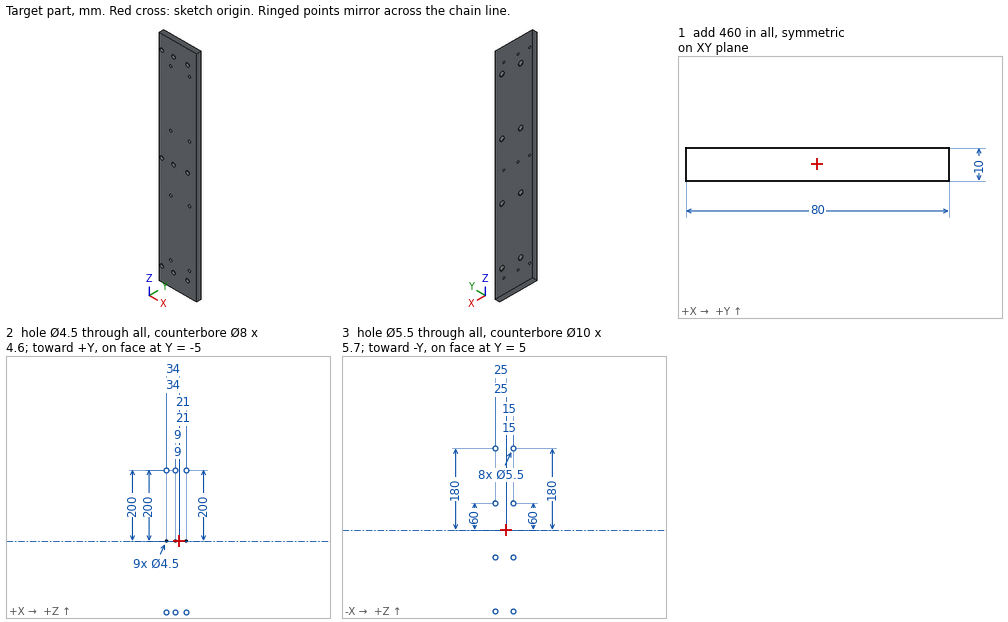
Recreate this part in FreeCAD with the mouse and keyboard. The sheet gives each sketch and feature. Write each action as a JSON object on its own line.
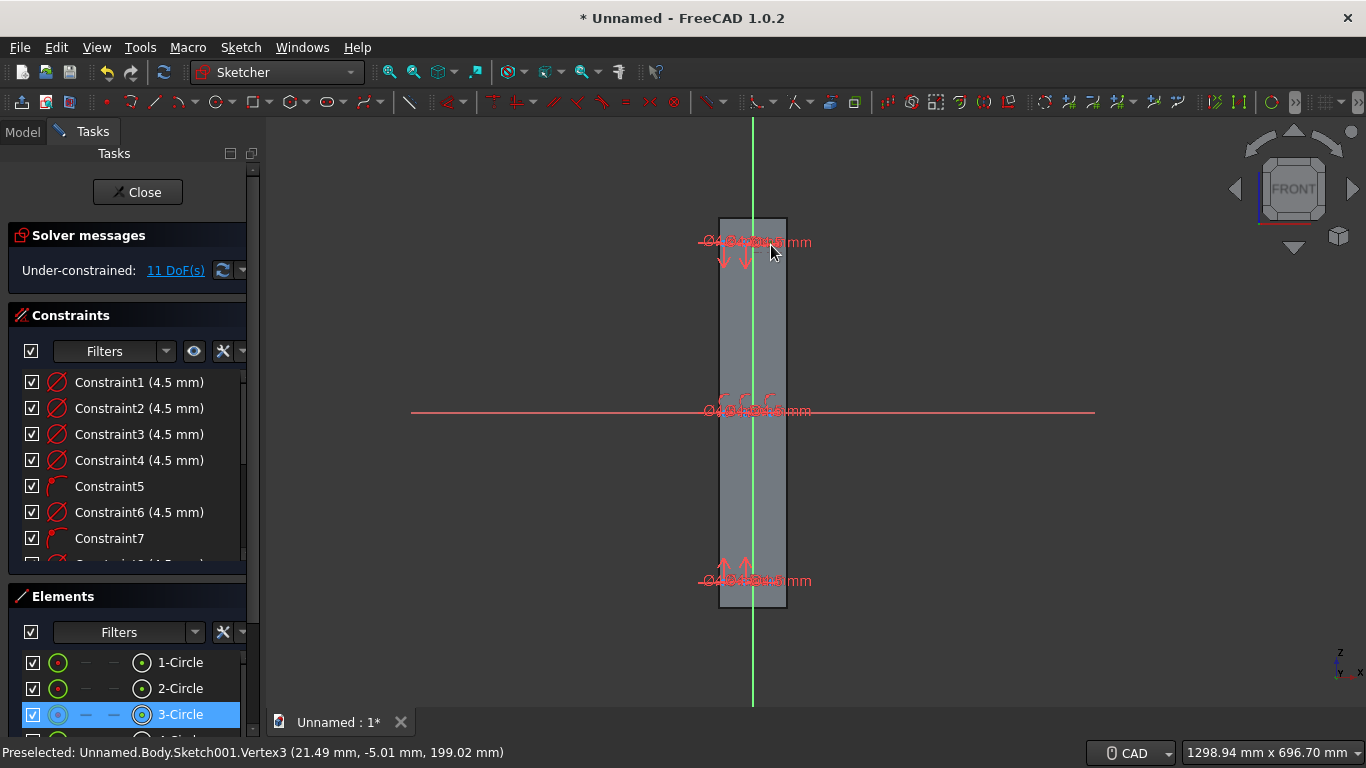
{"action": "left_click", "coordinate": [771, 583]}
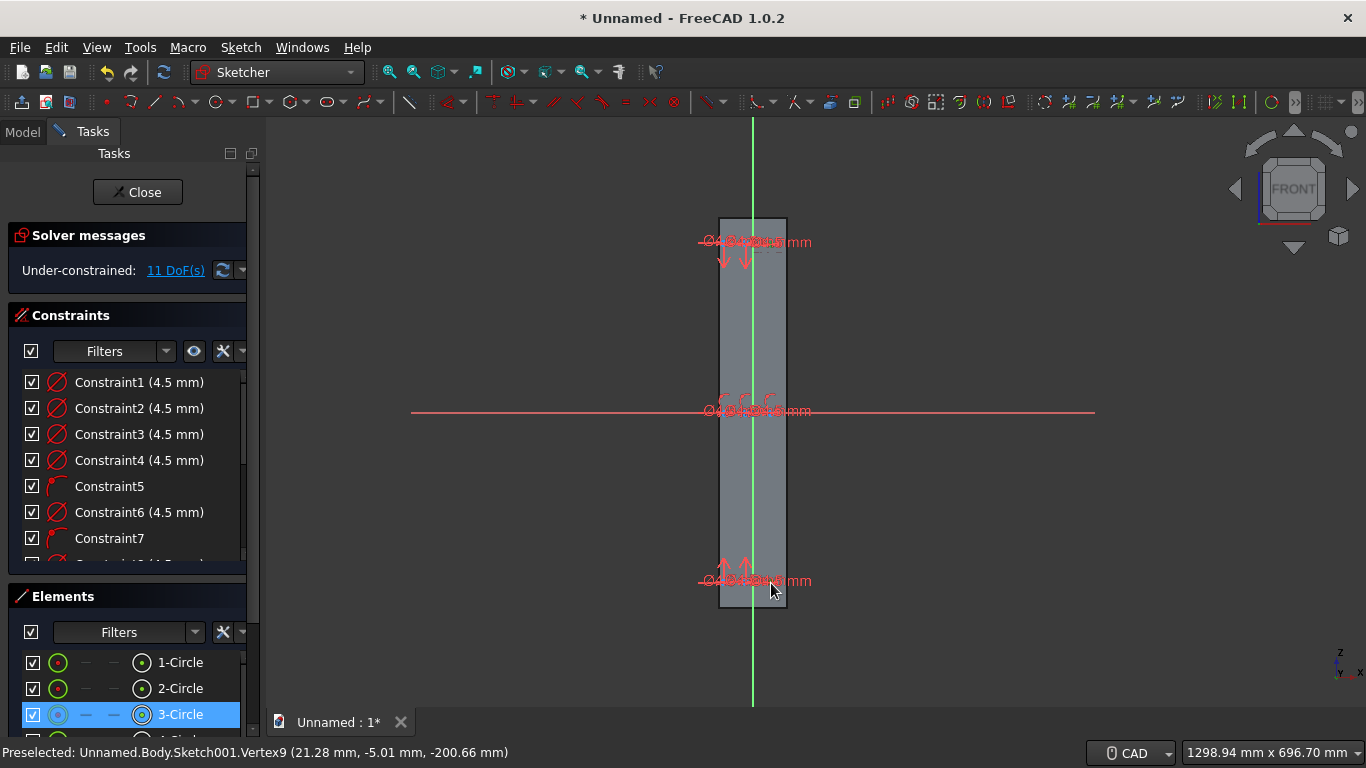
{"action": "left_click", "coordinate": [424, 413]}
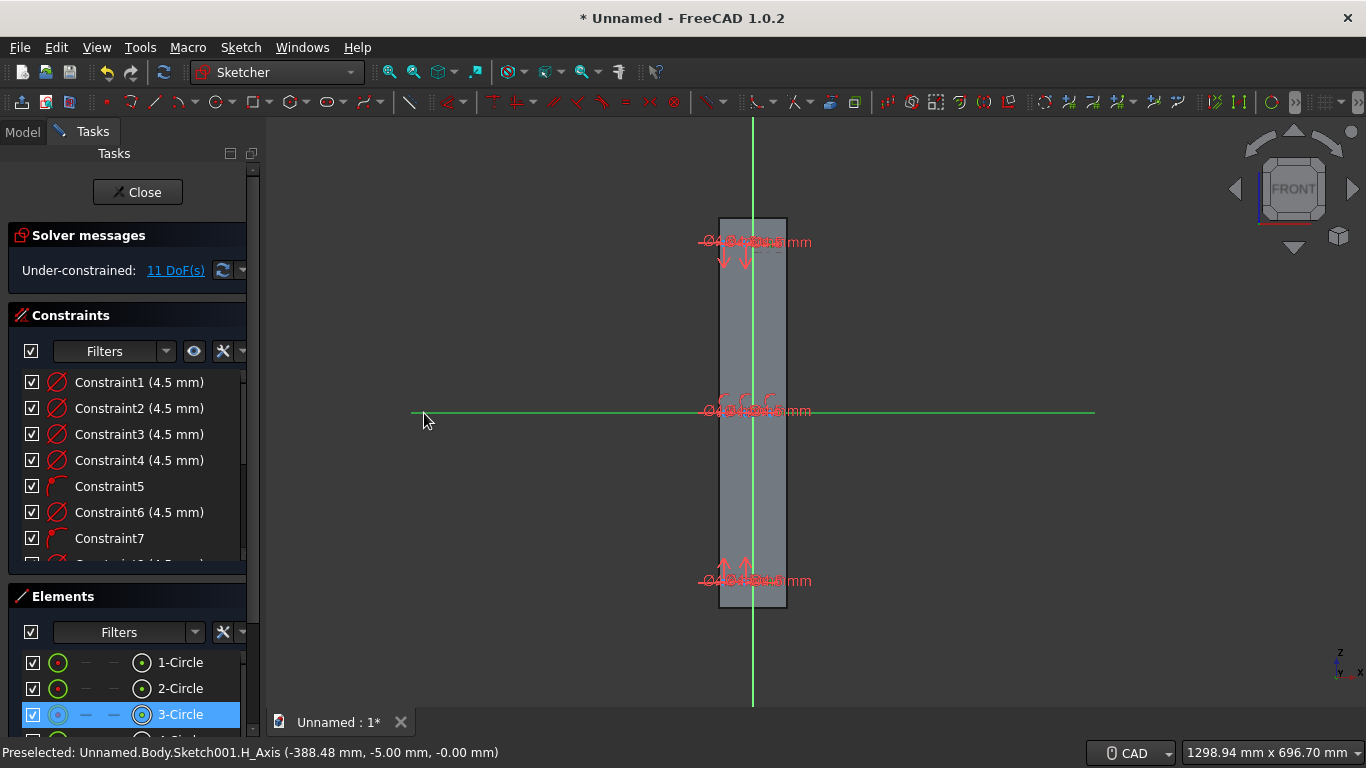
{"action": "key", "text": "s"}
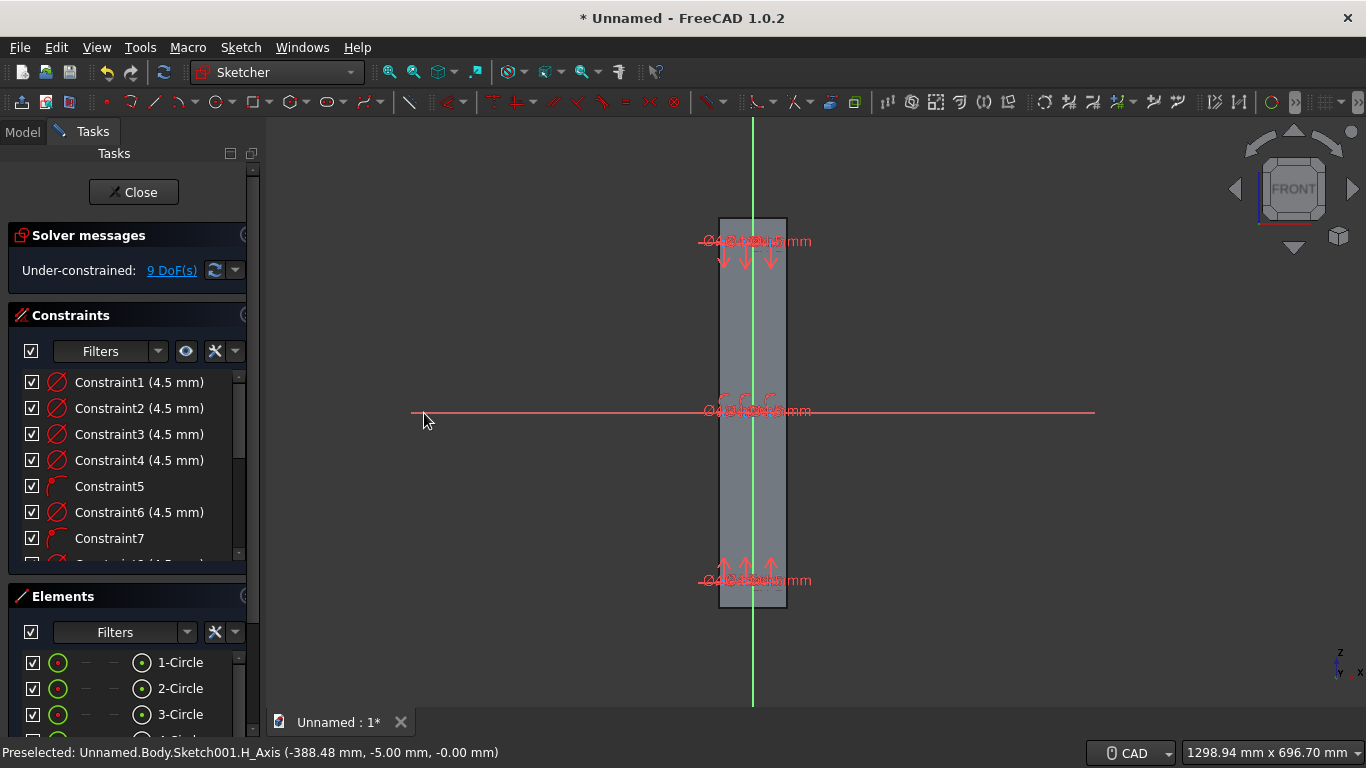
{"action": "key", "text": "d"}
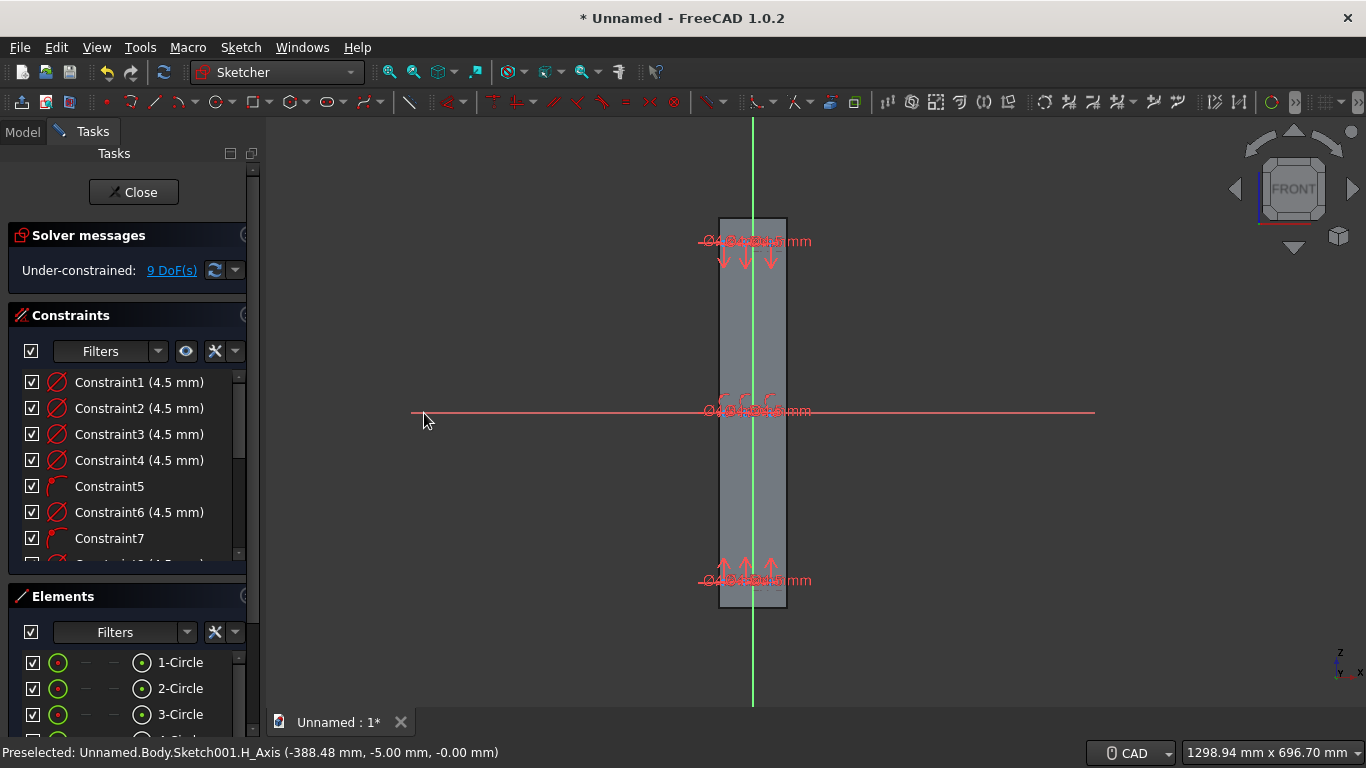
{"action": "scroll", "coordinate": [746, 244], "scroll_direction": "up", "scroll_amount": 9}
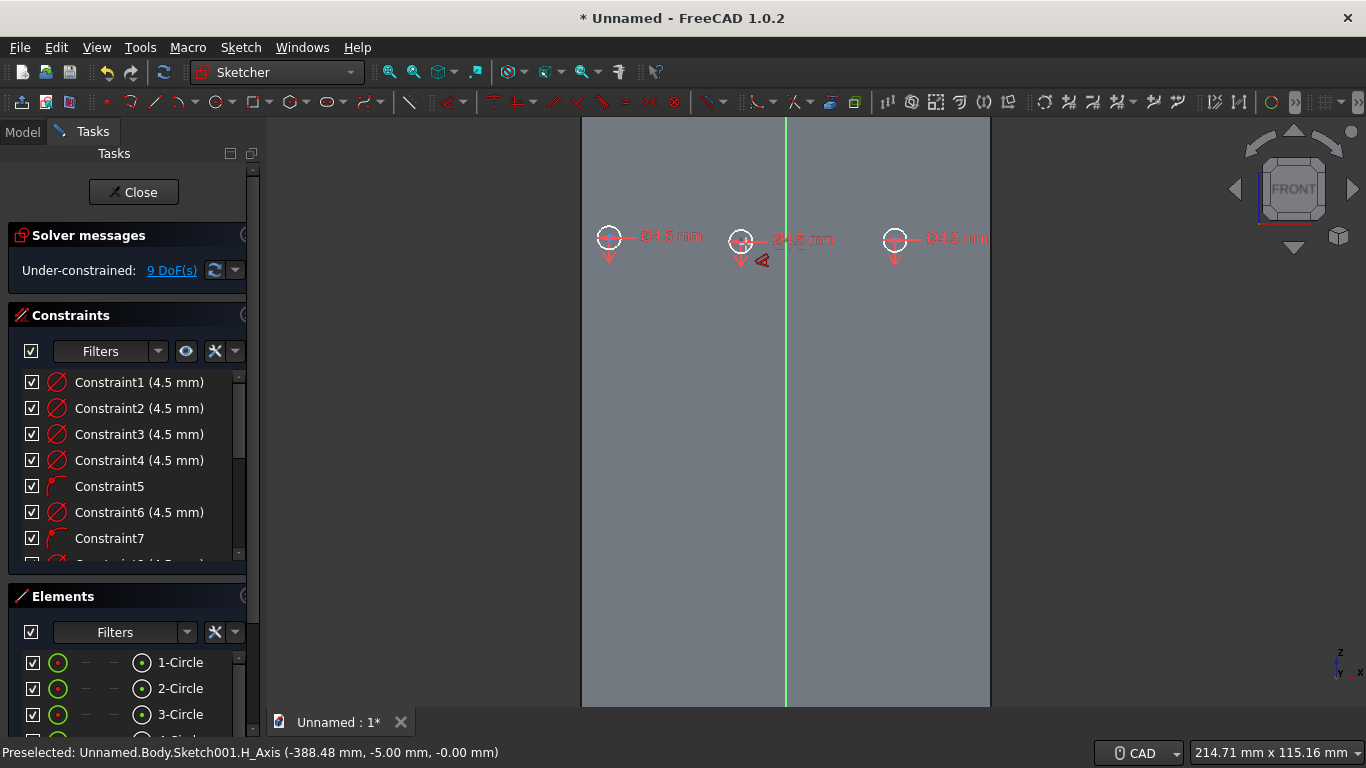
{"action": "left_click", "coordinate": [741, 242]}
{"action": "left_click", "coordinate": [763, 208]}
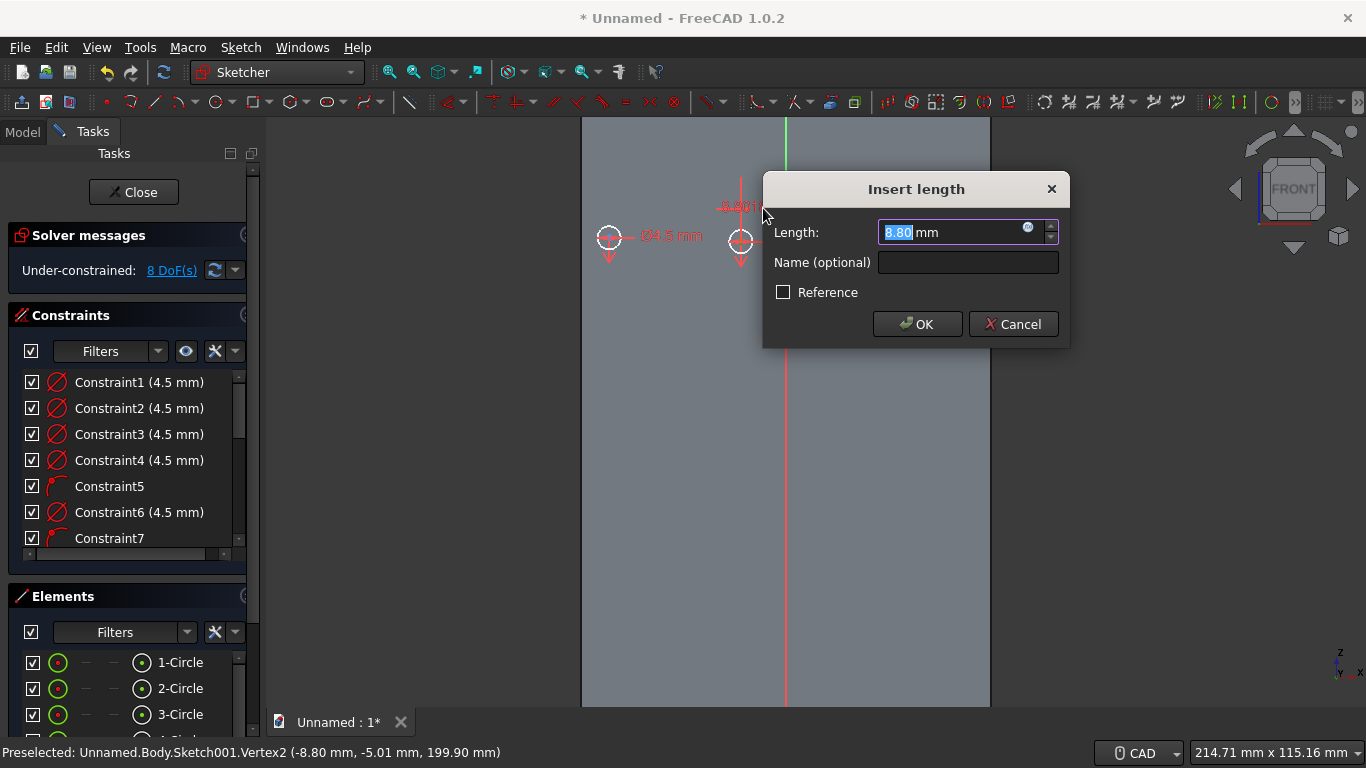
{"action": "type", "text": "9"}
{"action": "key", "text": "Return"}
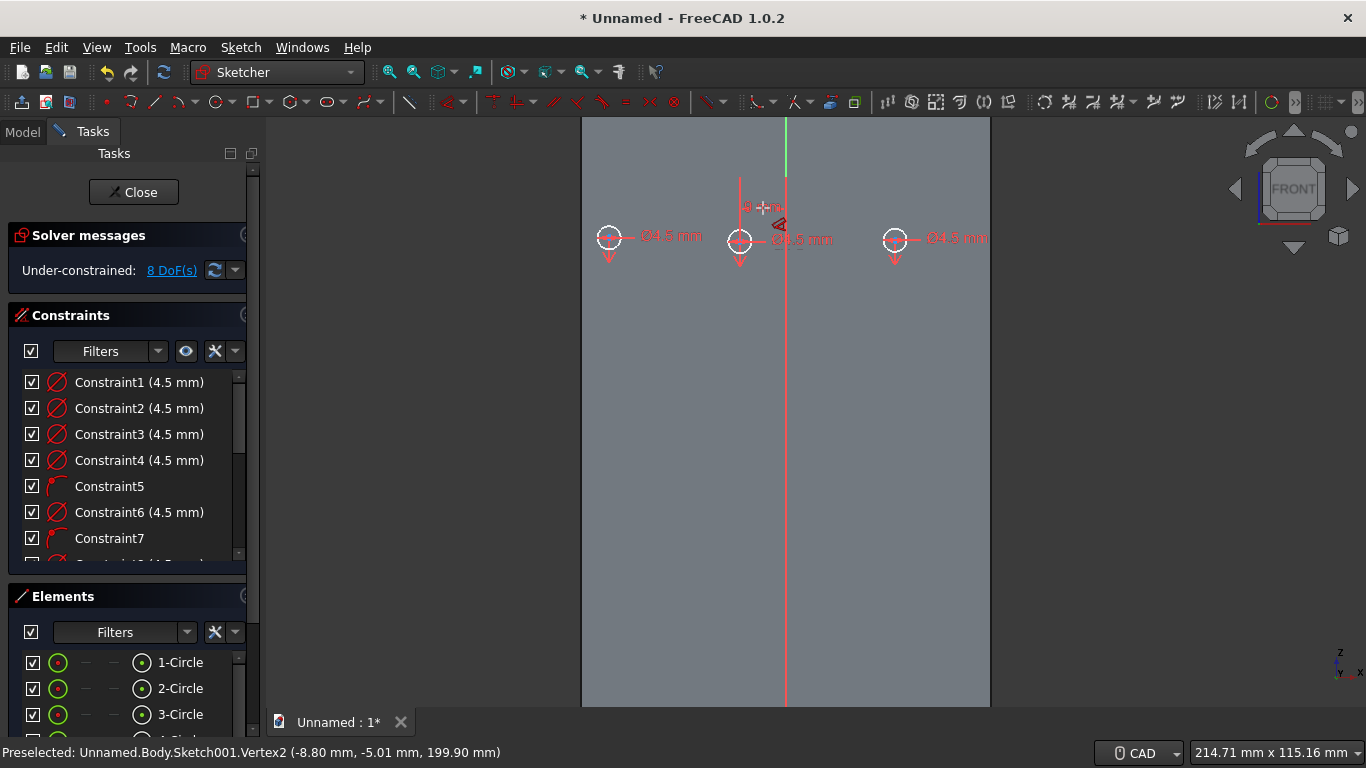
{"action": "scroll", "coordinate": [746, 243], "scroll_direction": "down", "scroll_amount": 9}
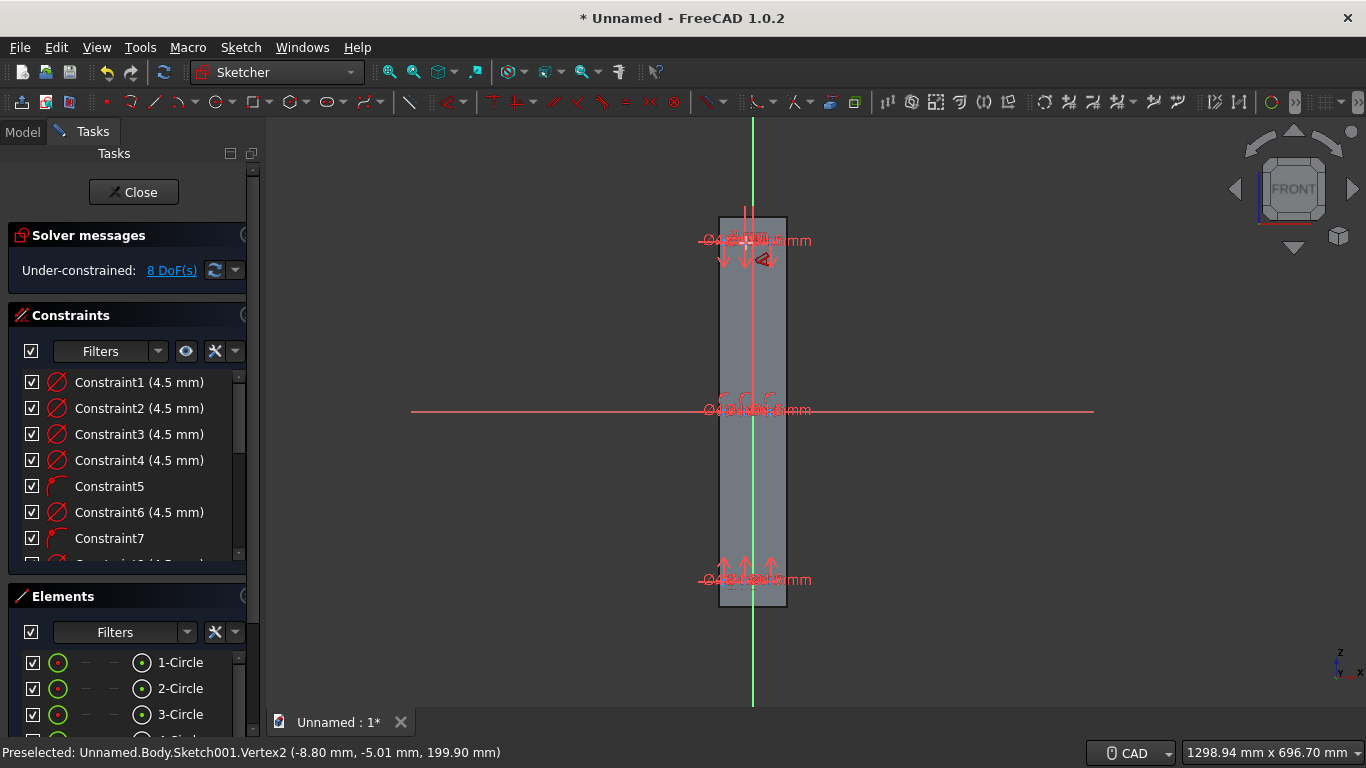
{"action": "scroll", "coordinate": [745, 412], "scroll_direction": "up", "scroll_amount": 9}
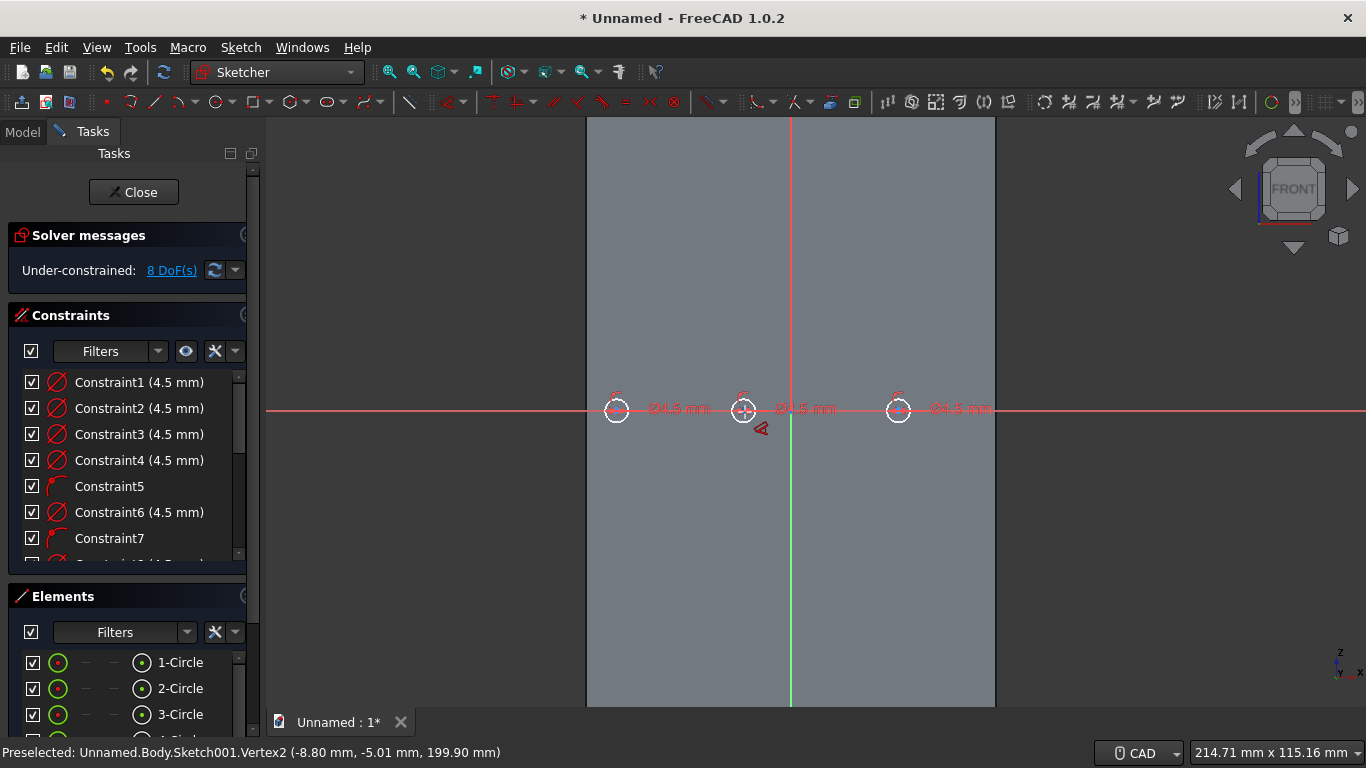
{"action": "left_click", "coordinate": [744, 411]}
{"action": "left_click", "coordinate": [767, 445]}